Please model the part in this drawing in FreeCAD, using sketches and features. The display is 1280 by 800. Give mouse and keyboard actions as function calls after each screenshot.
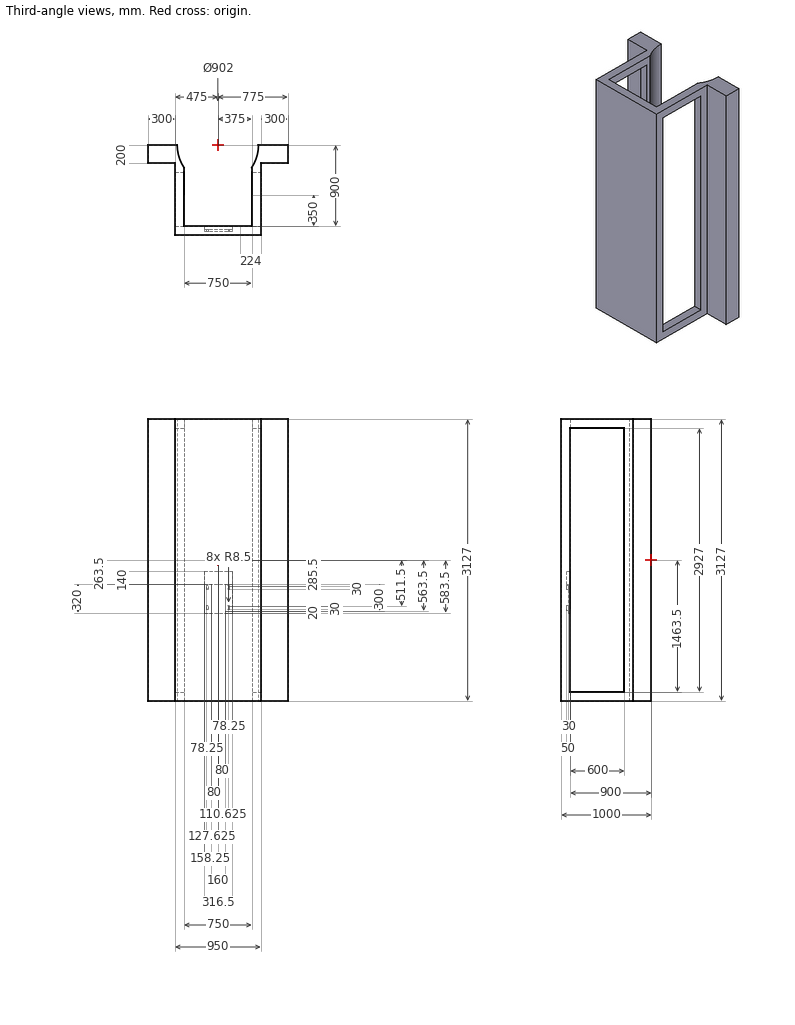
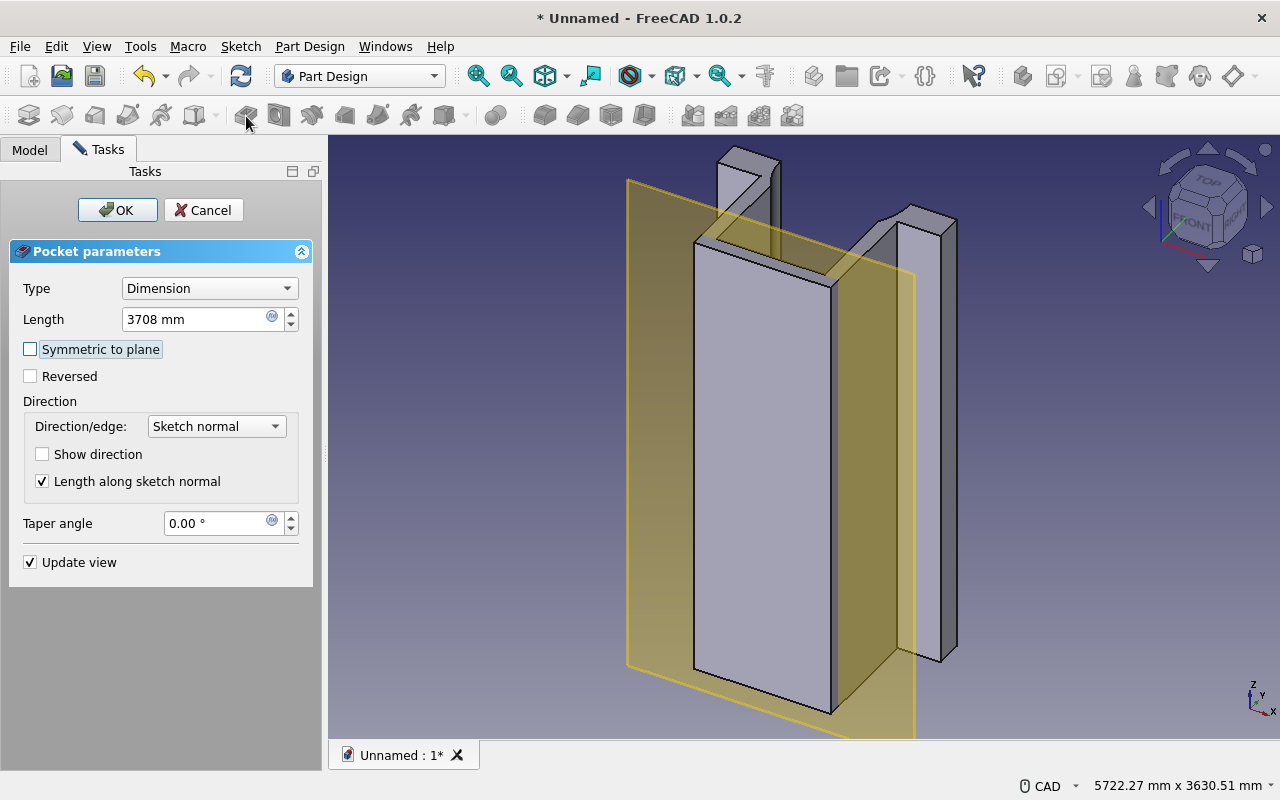
click(118, 210)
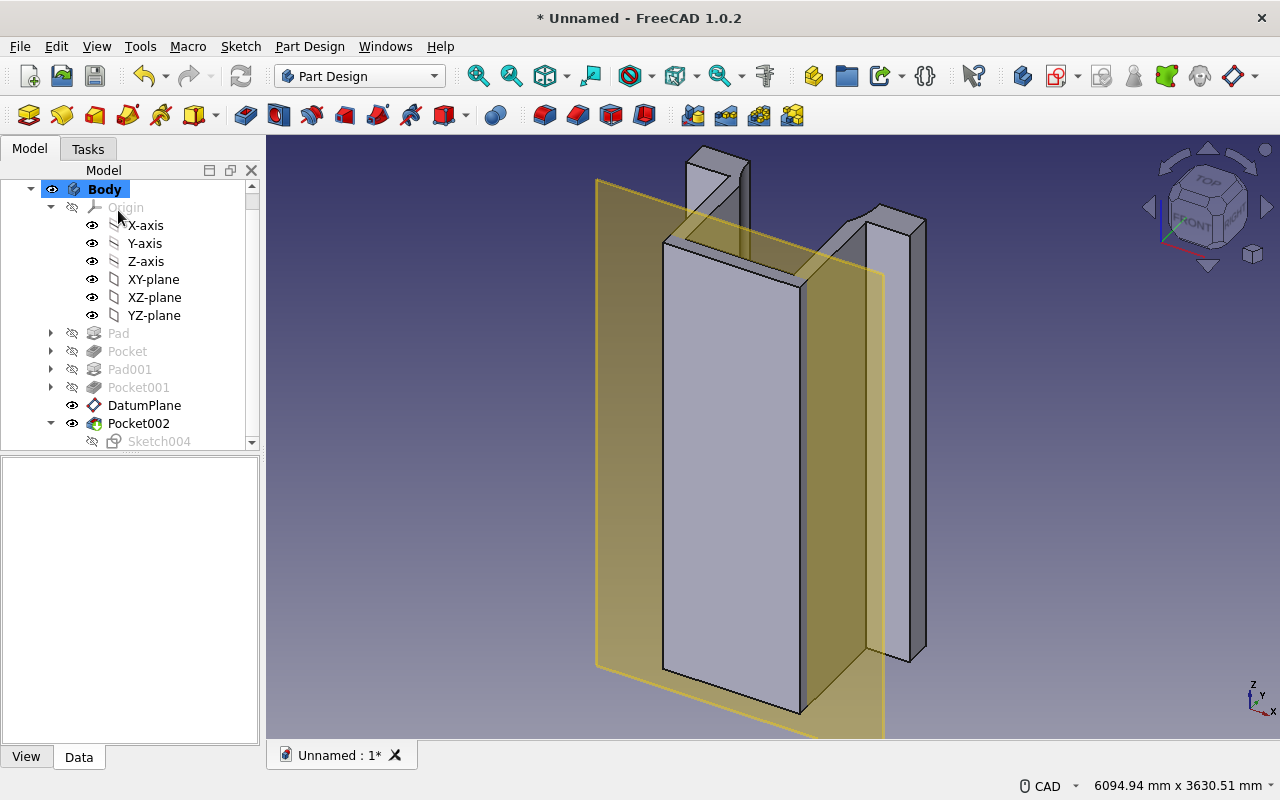
click(117, 405)
key(space)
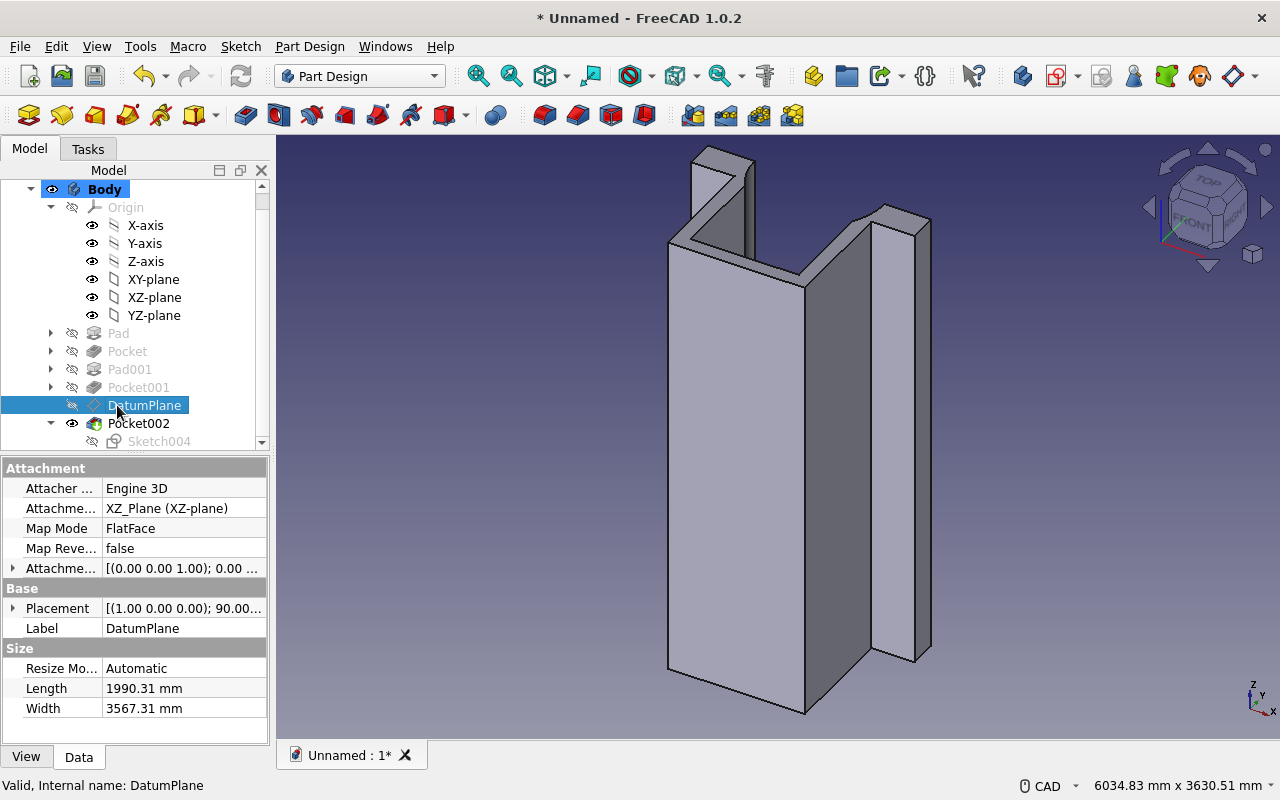
key(4)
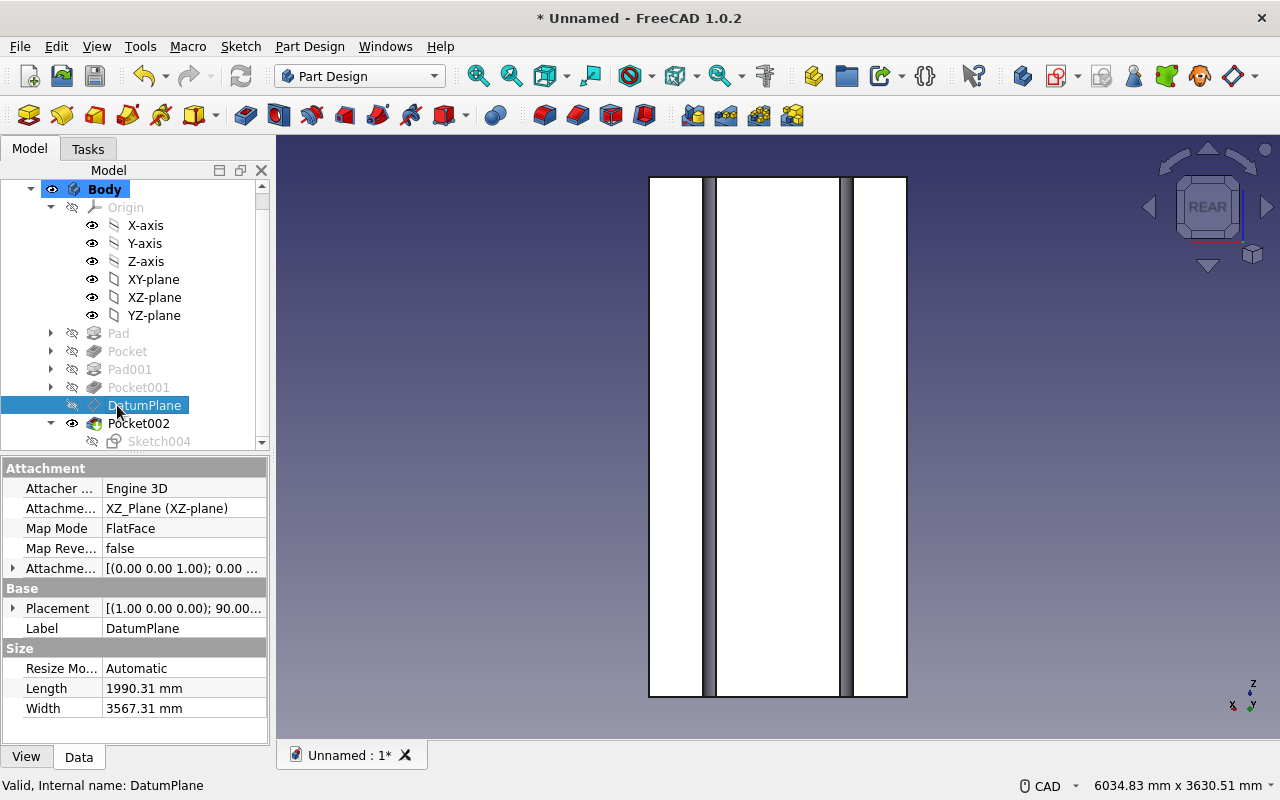
click(778, 287)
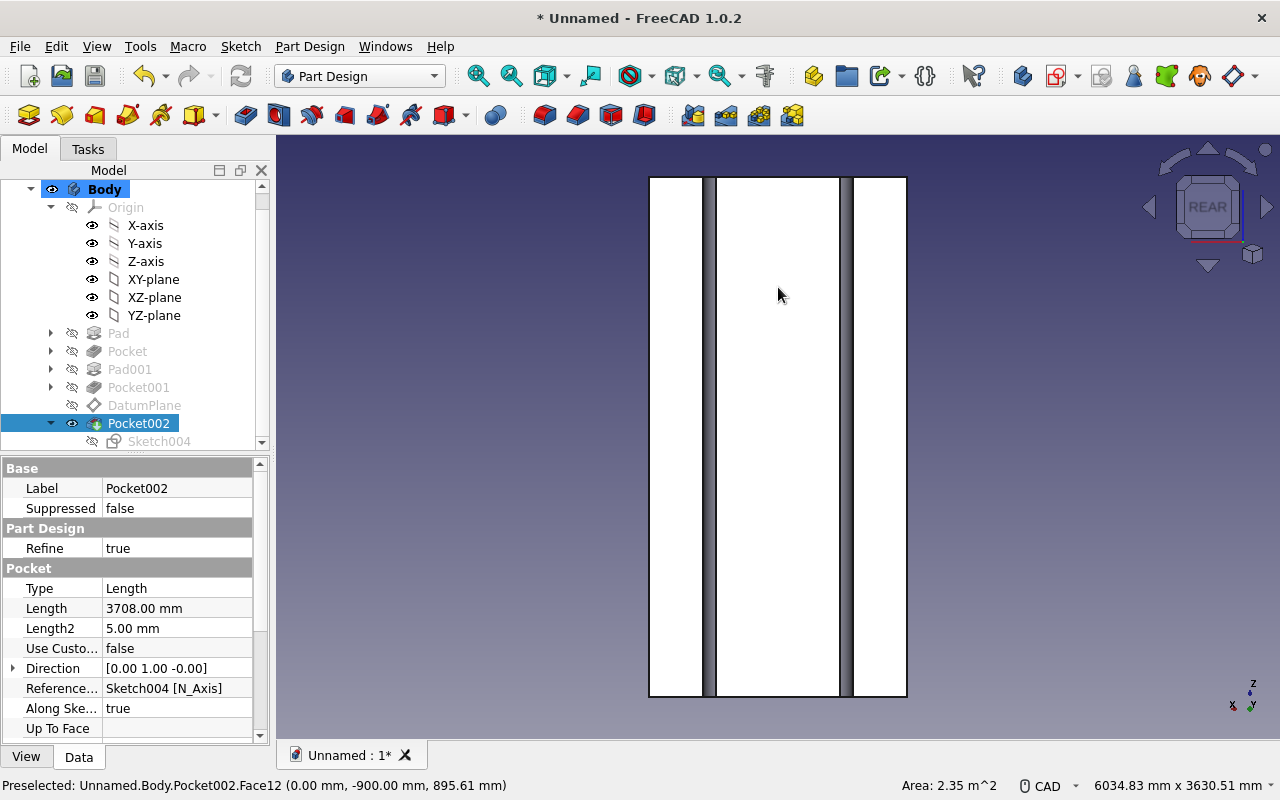
click(1056, 76)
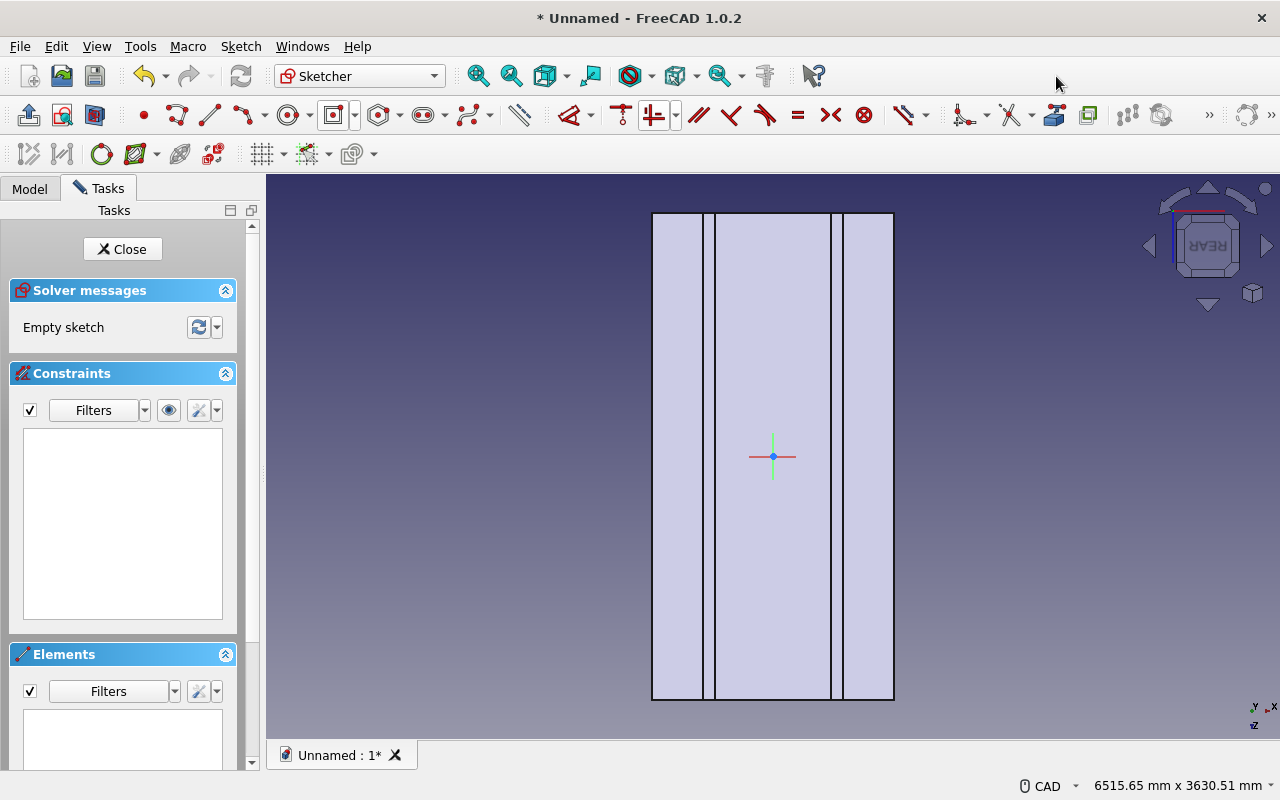
click(95, 116)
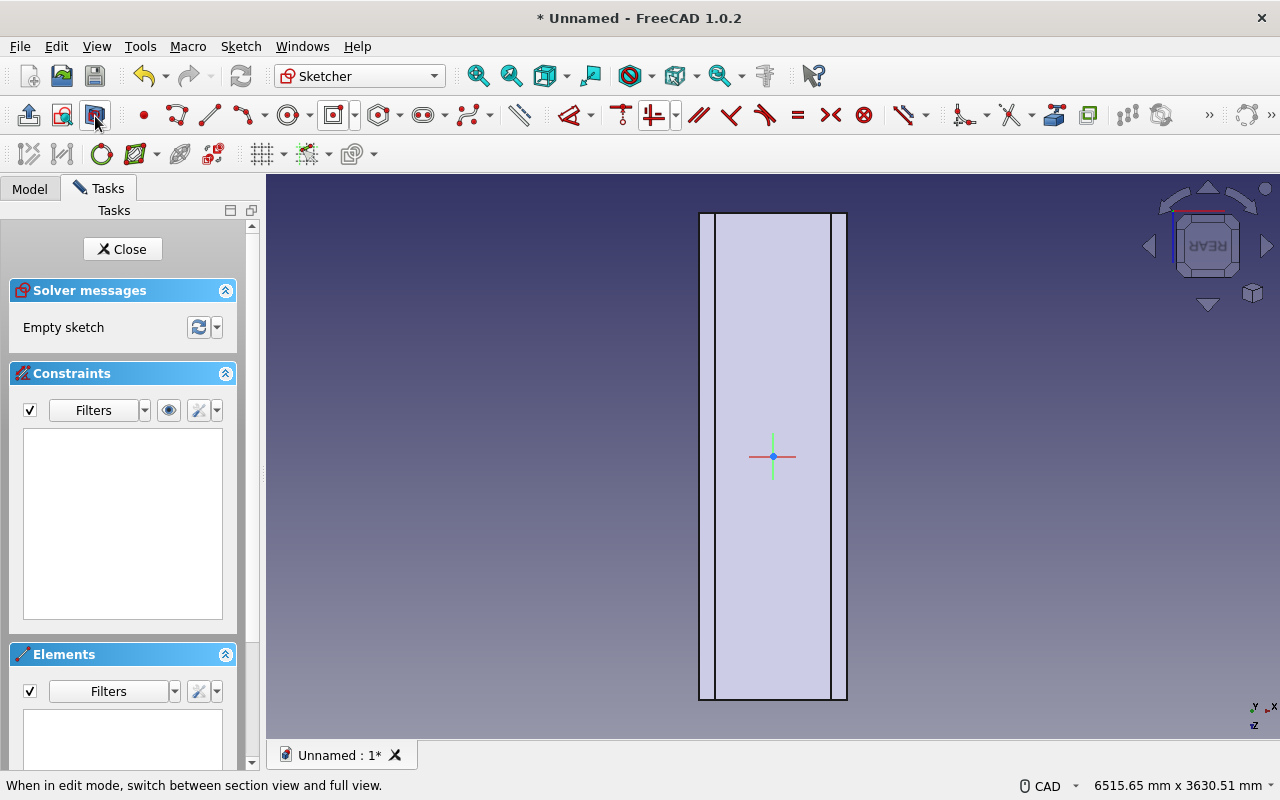
scroll(795, 400, up, 7)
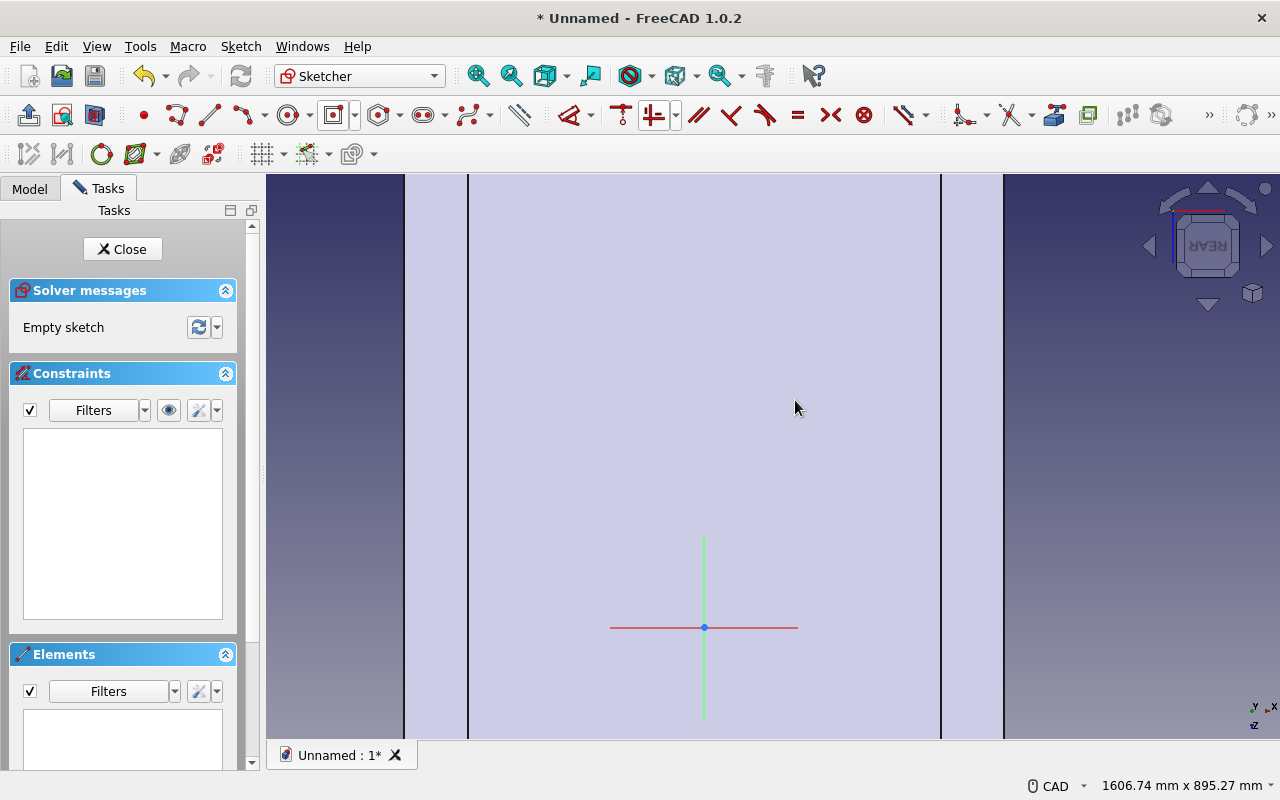
click(422, 116)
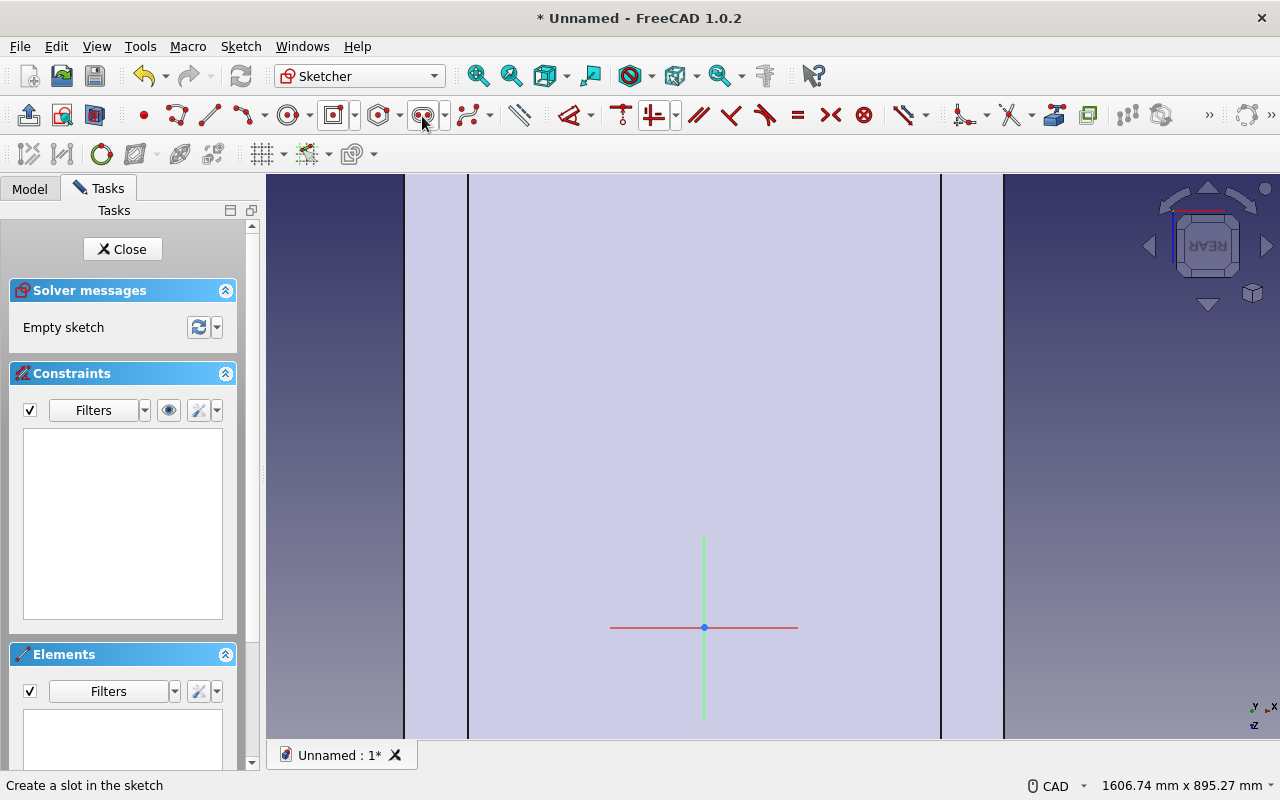
scroll(779, 305, up, 8)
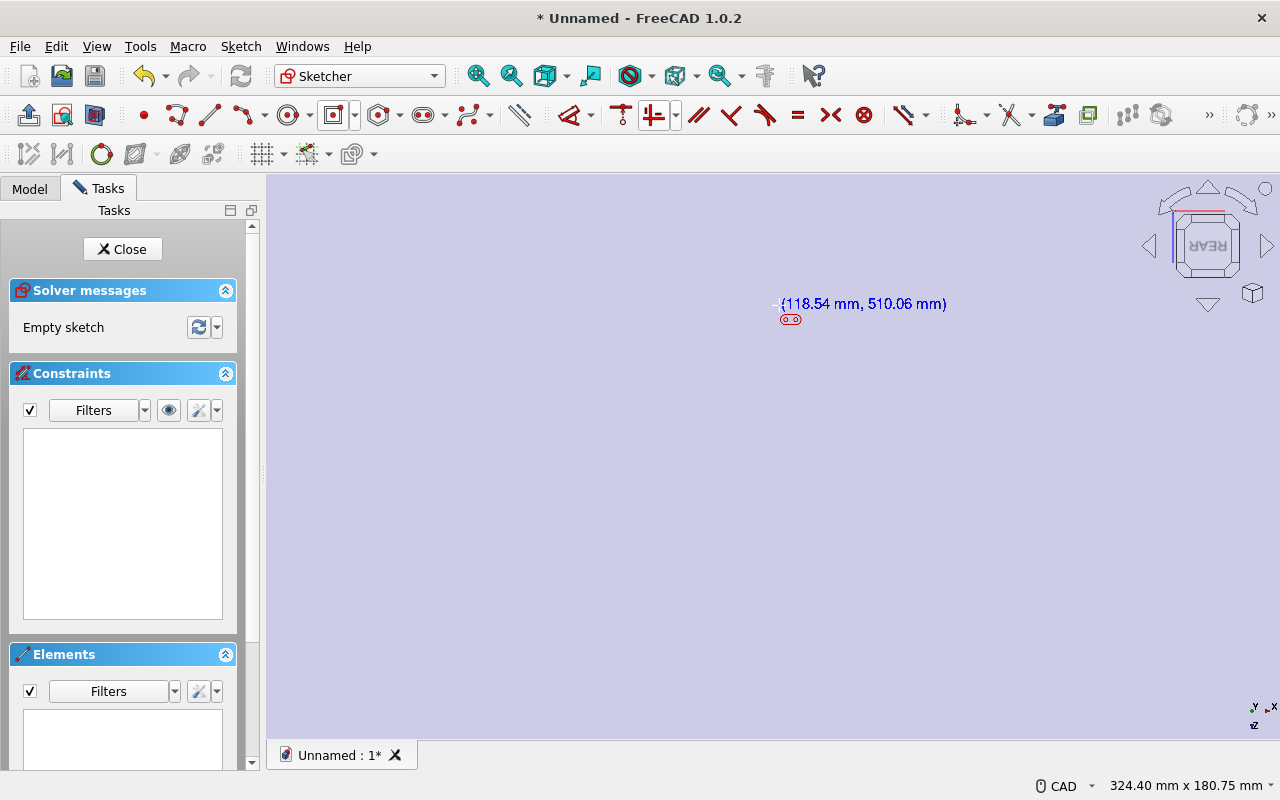
scroll(780, 308, down, 8)